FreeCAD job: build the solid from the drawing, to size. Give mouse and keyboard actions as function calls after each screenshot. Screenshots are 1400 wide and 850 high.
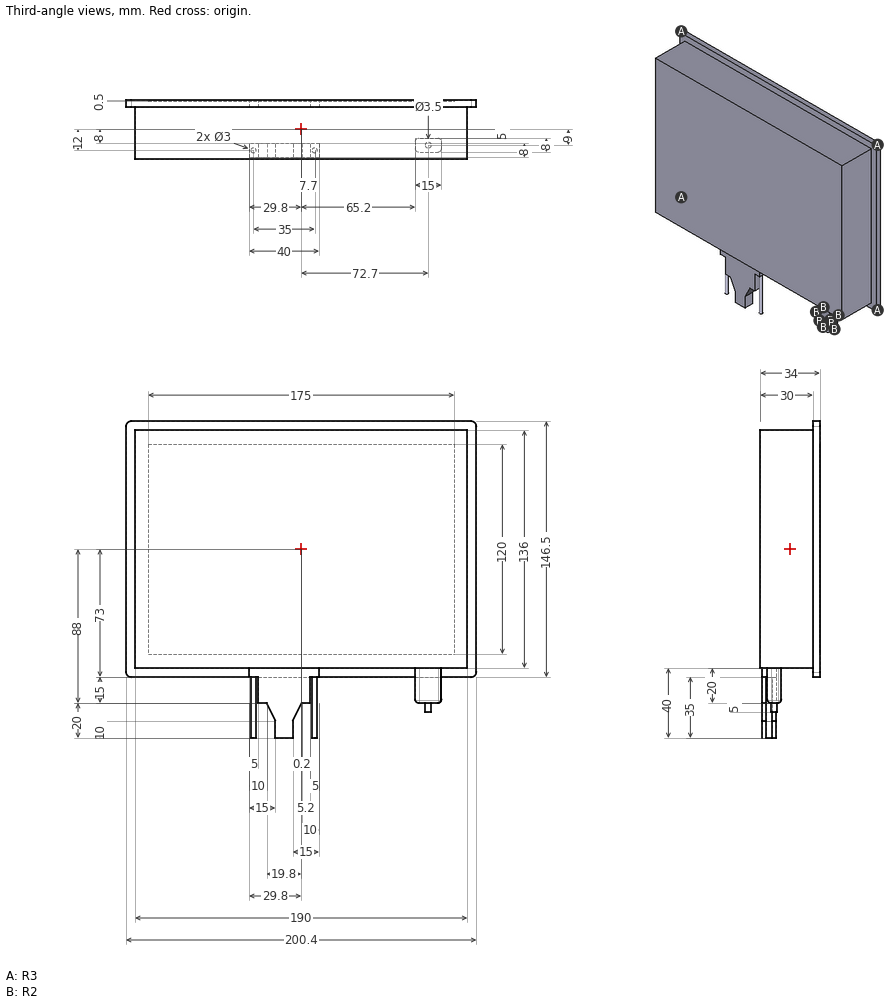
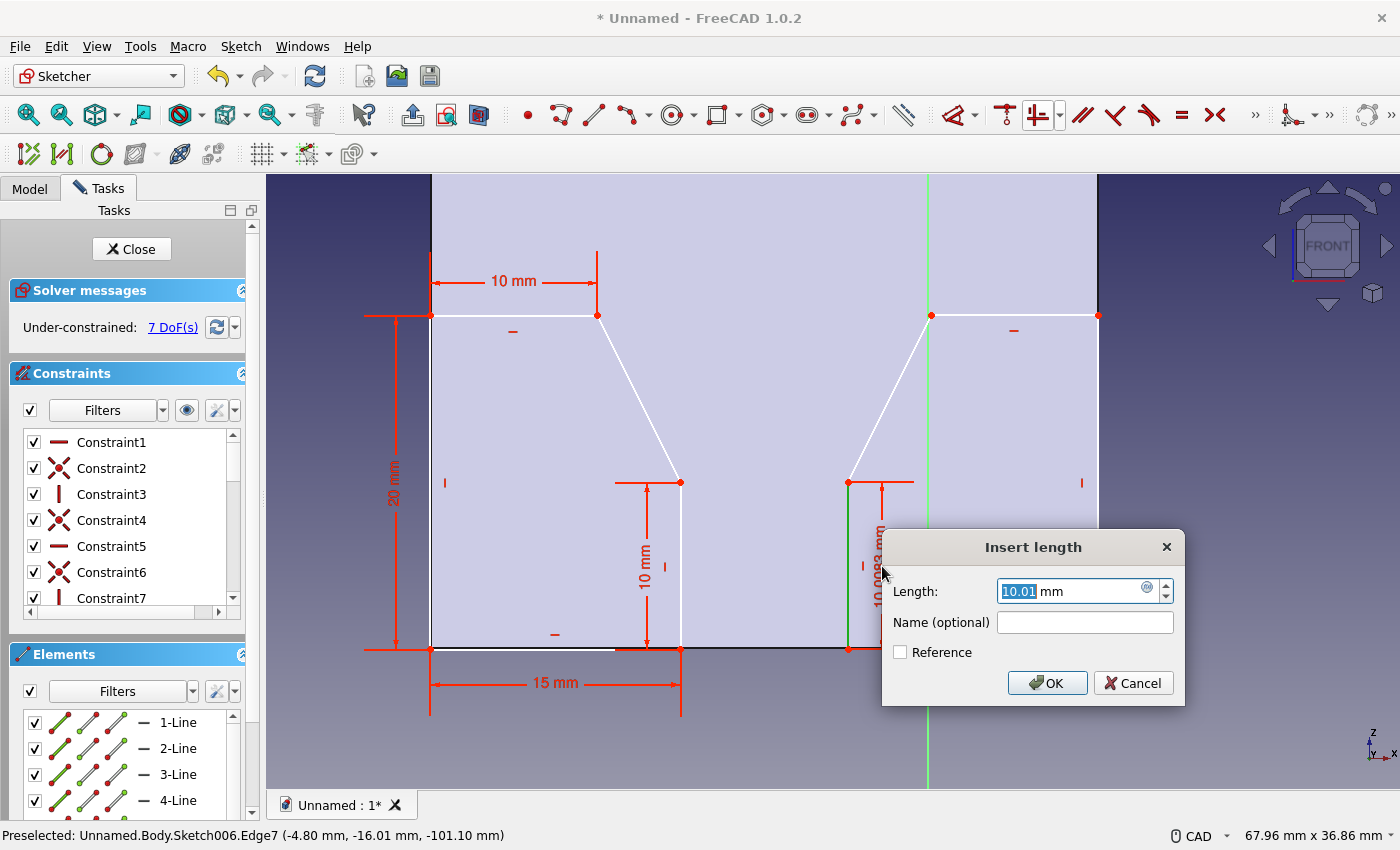
text(10)
key(Return)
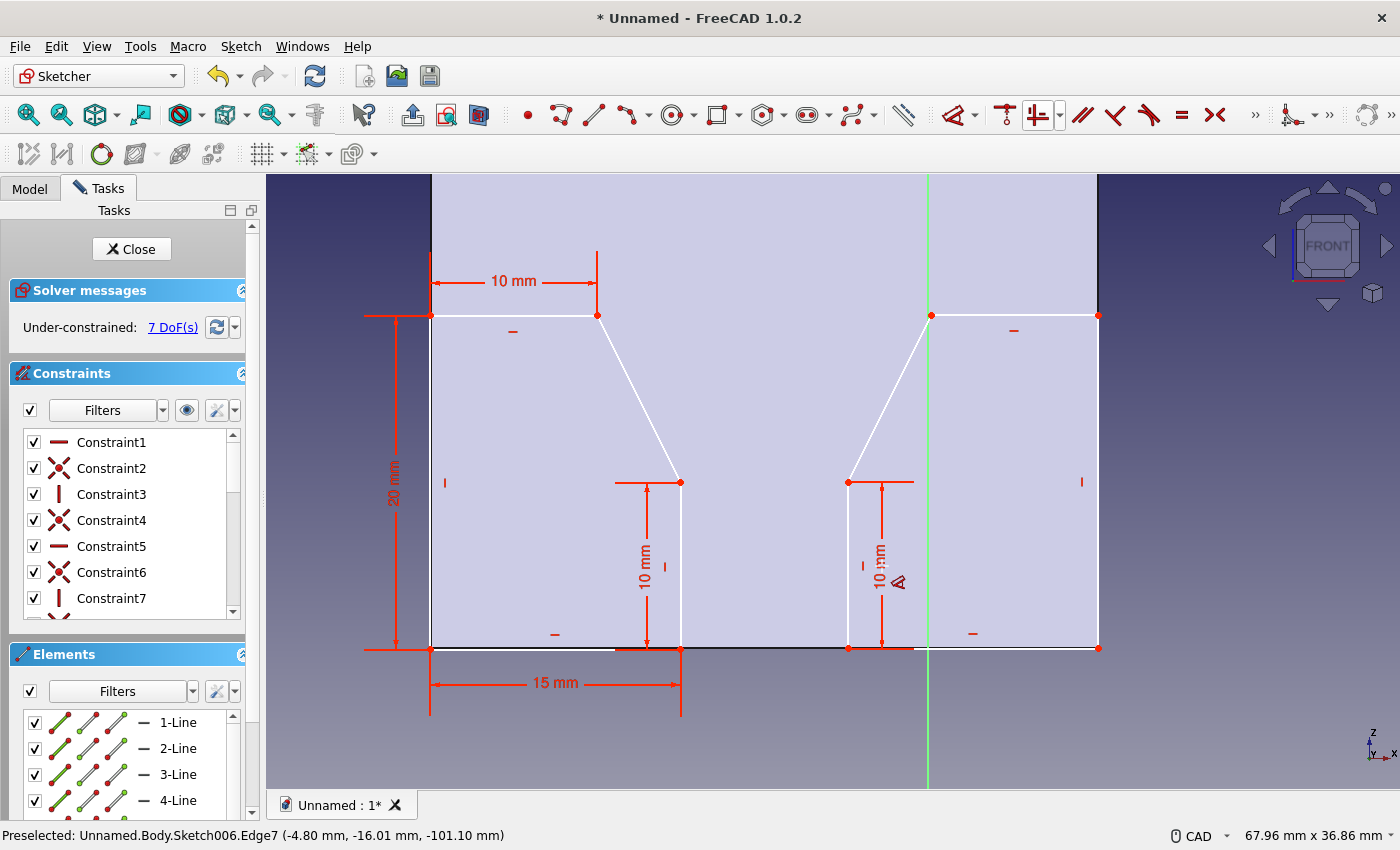
click(1023, 649)
click(973, 683)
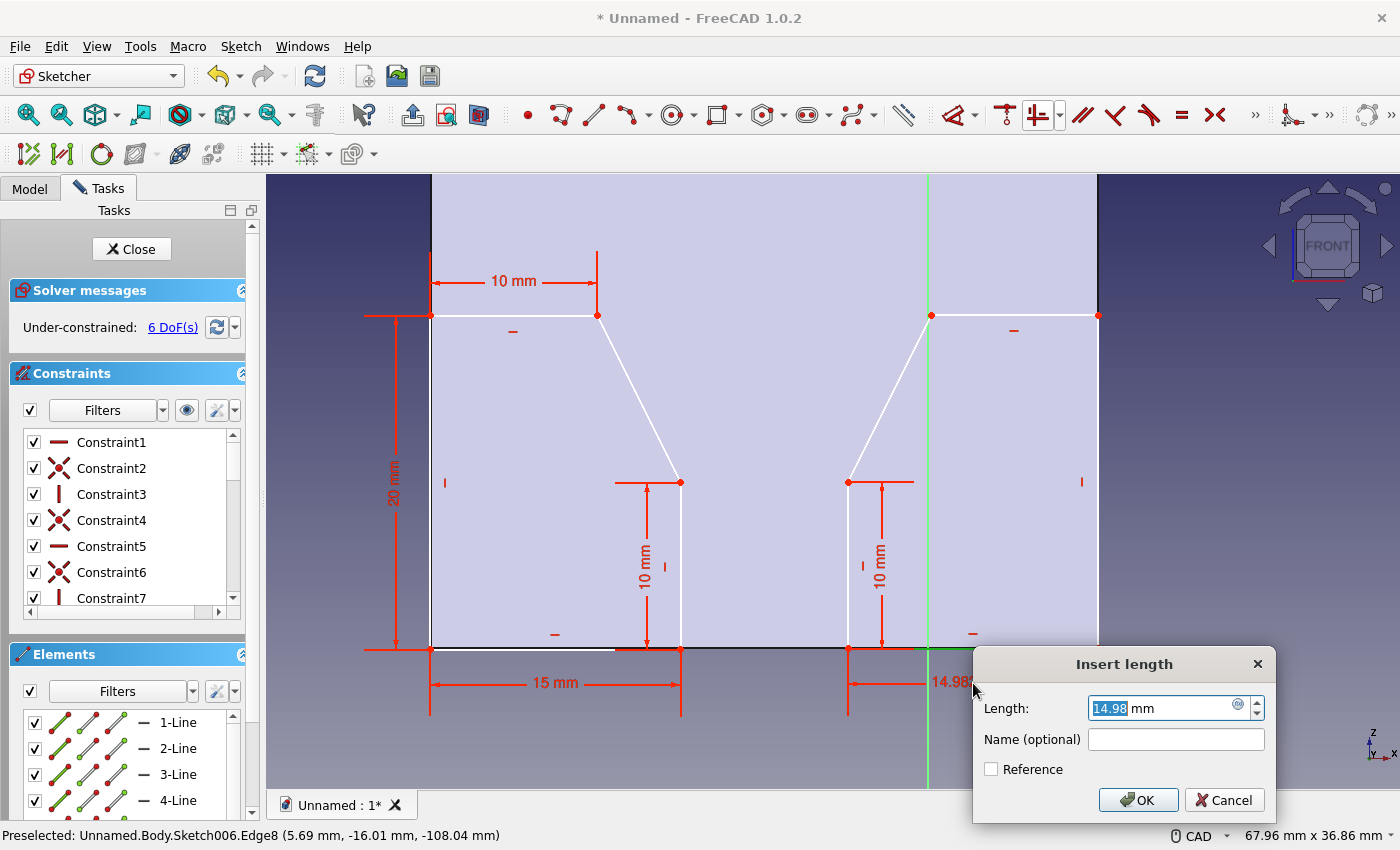
text(15)
key(Return)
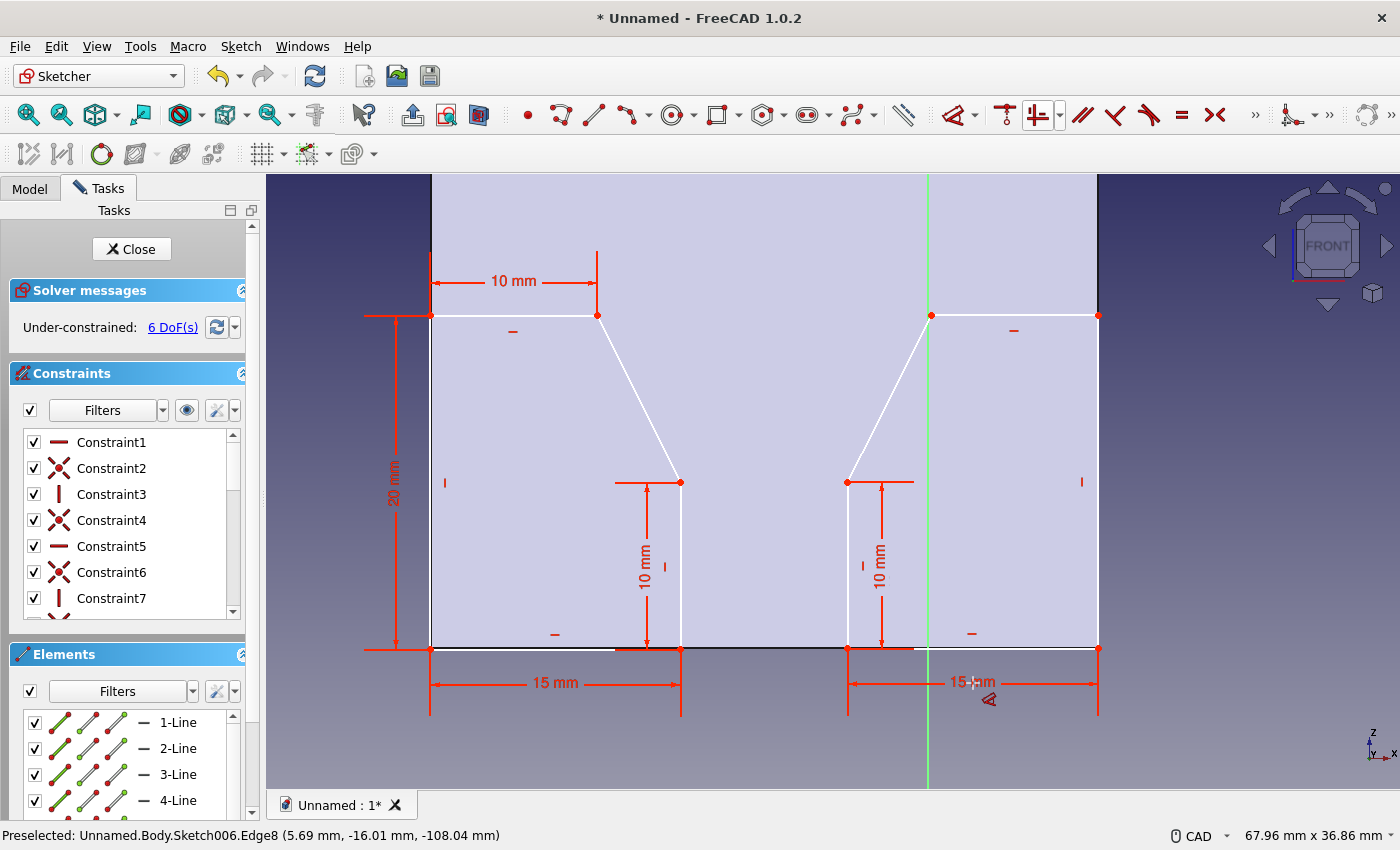
click(1098, 549)
click(1132, 482)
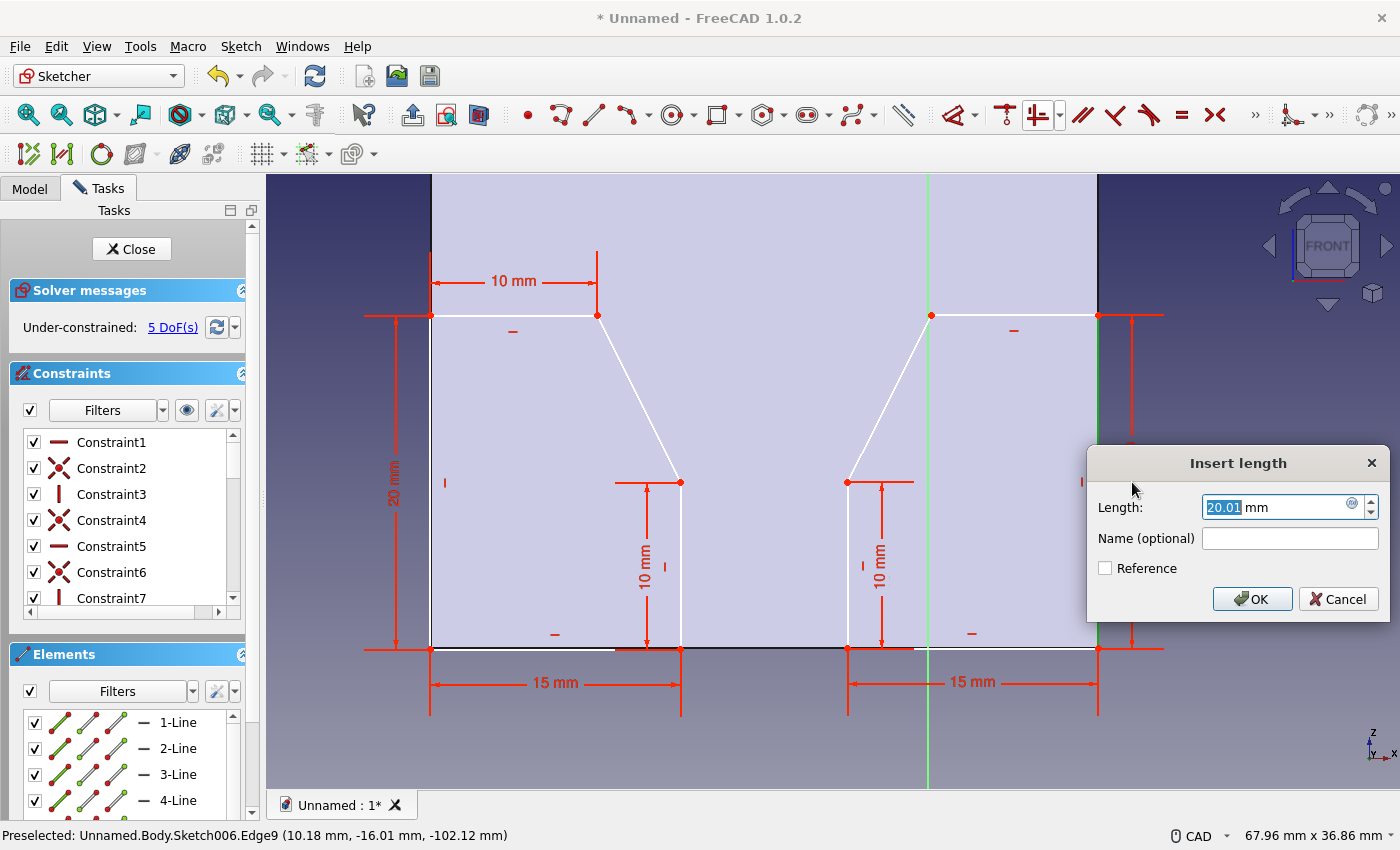
text(20)
key(Return)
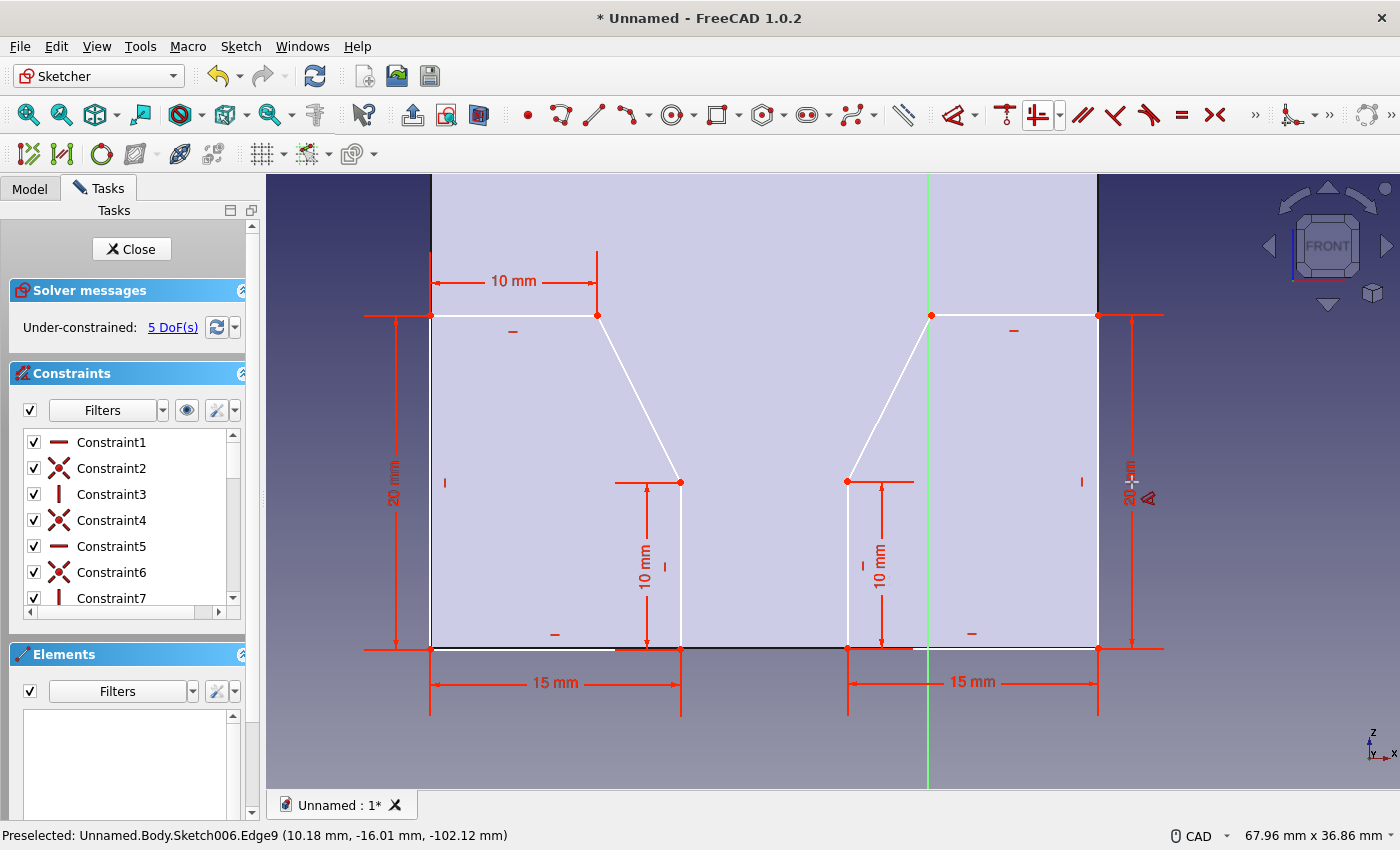
click(1048, 315)
click(1015, 281)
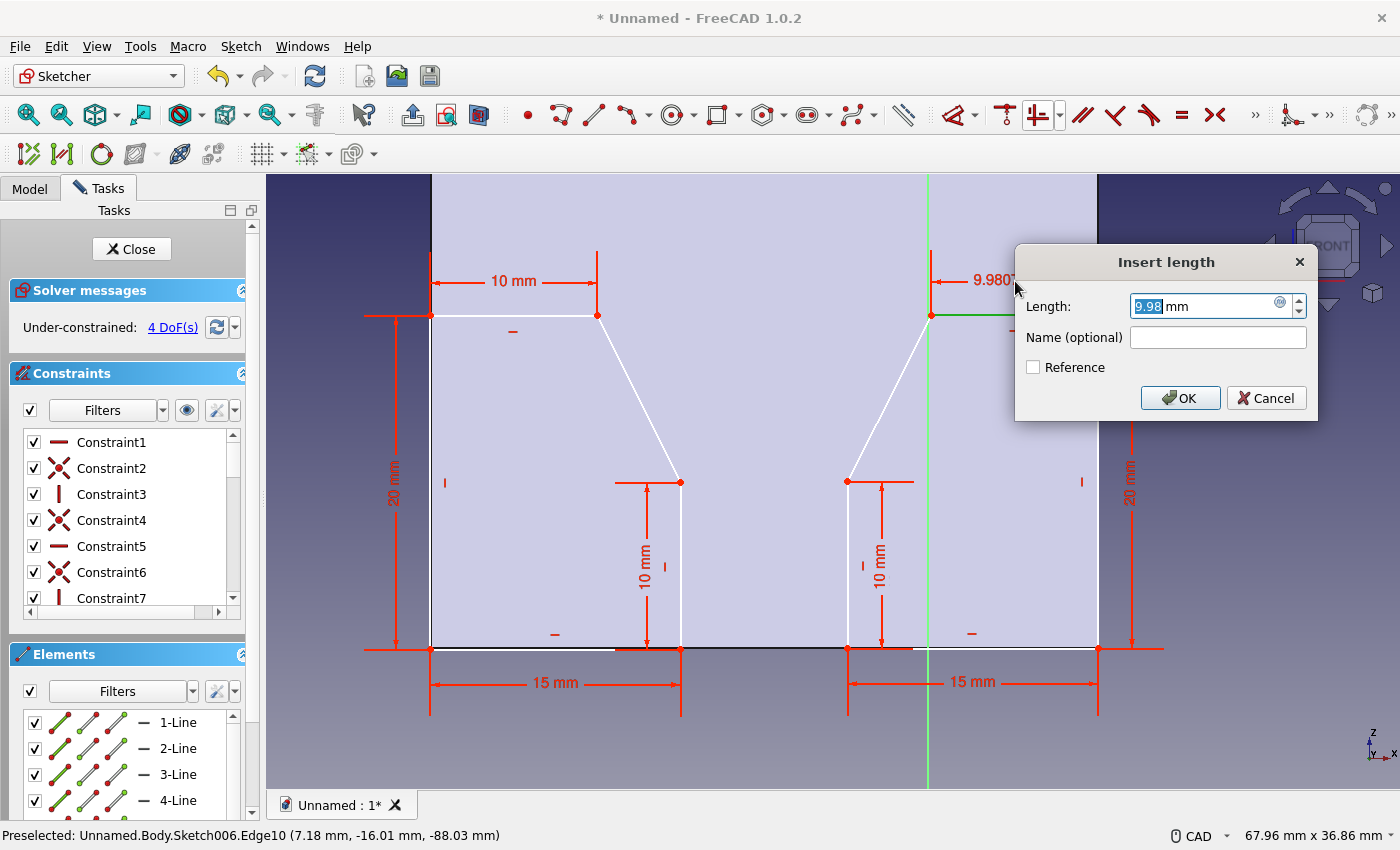
text(10)
key(Return)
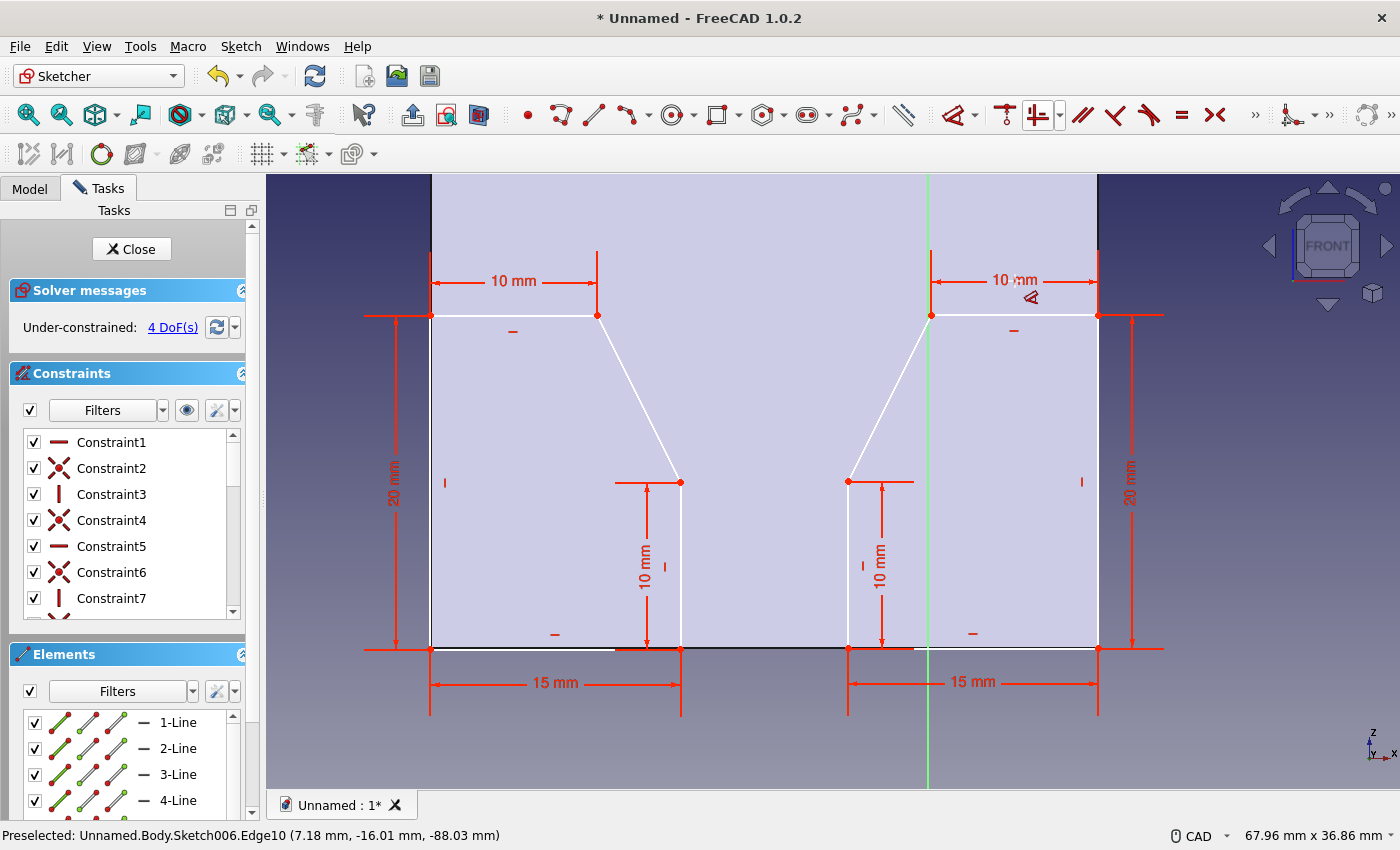
click(597, 316)
click(563, 259)